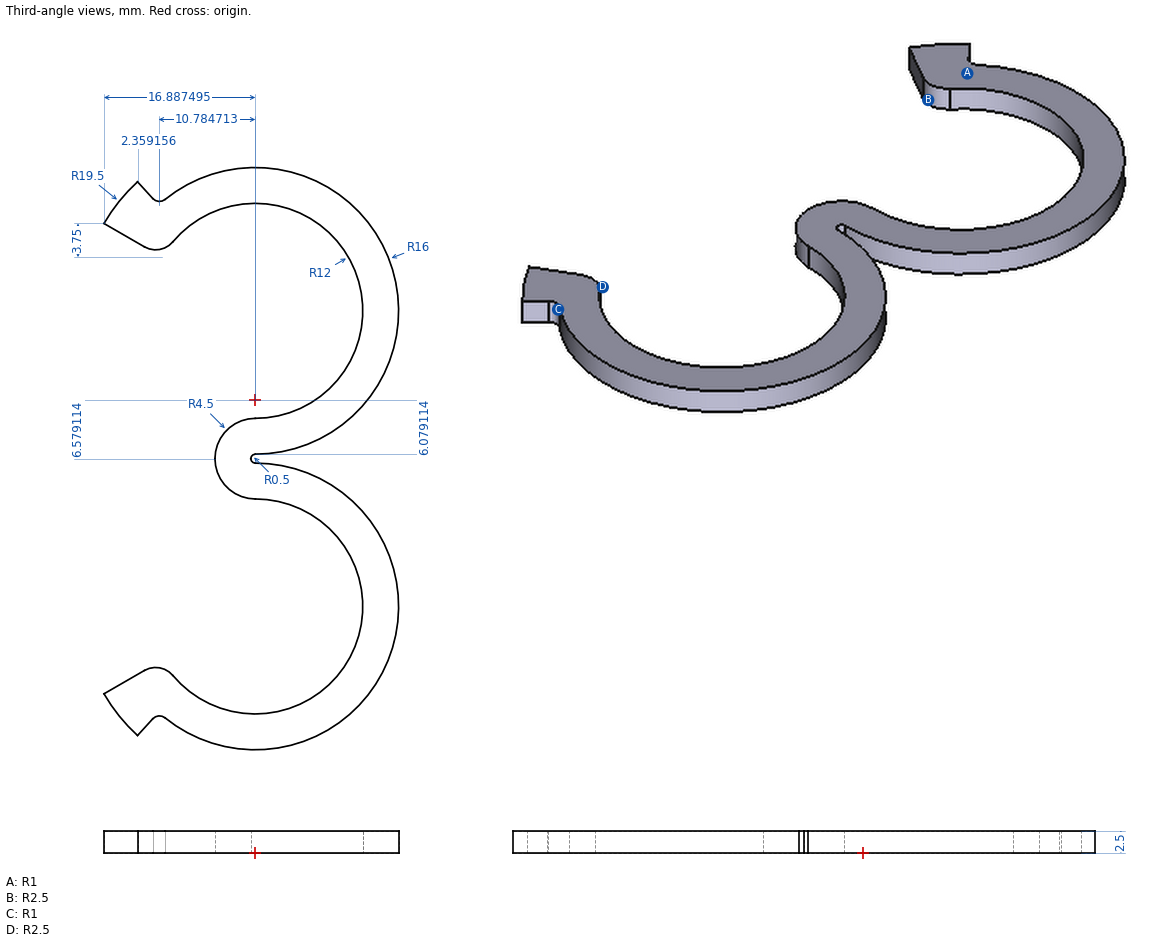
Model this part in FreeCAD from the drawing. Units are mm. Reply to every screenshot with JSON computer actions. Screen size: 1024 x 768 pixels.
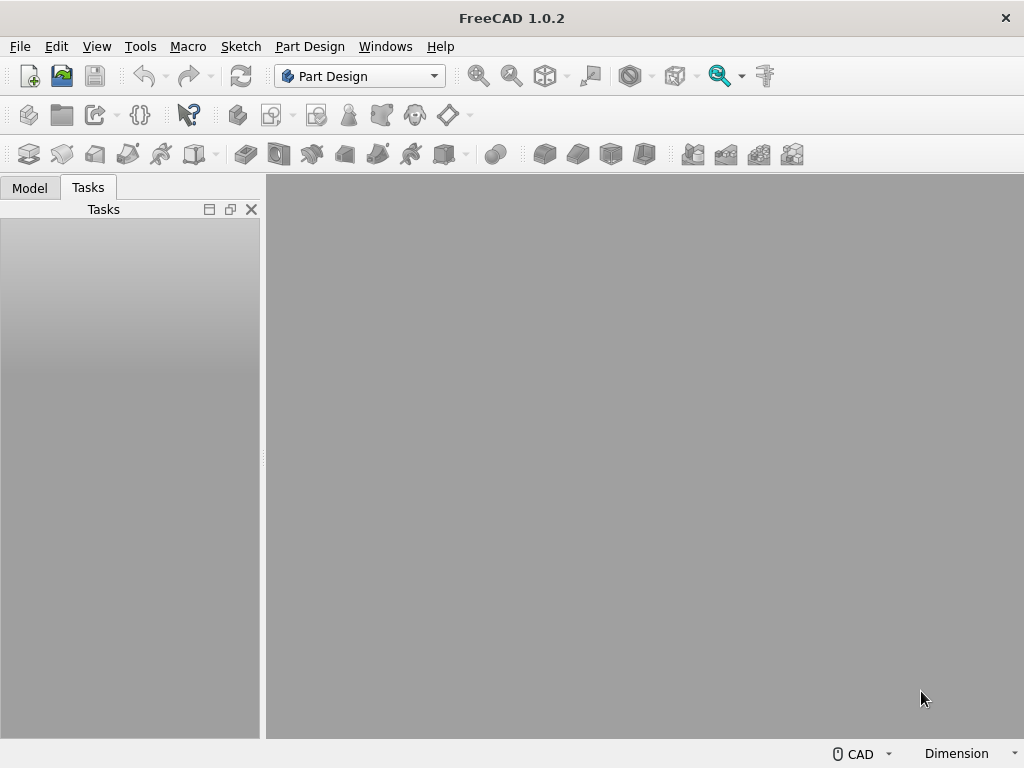
{"action": "left_click", "coordinate": [29, 76]}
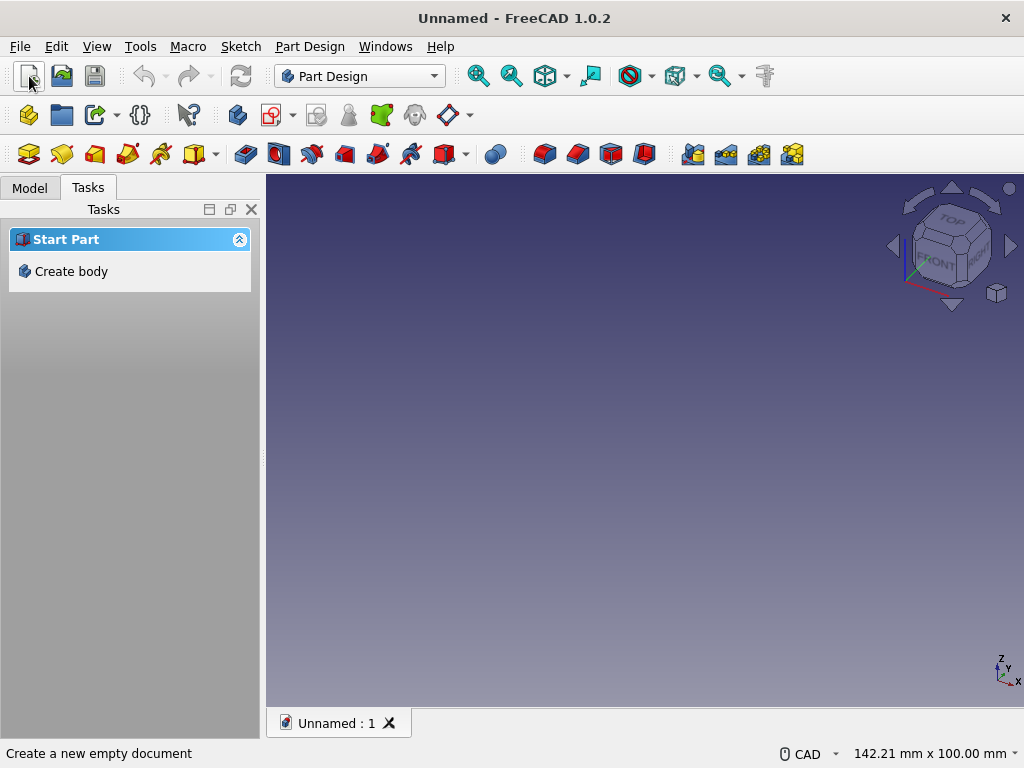
{"action": "left_click", "coordinate": [270, 116]}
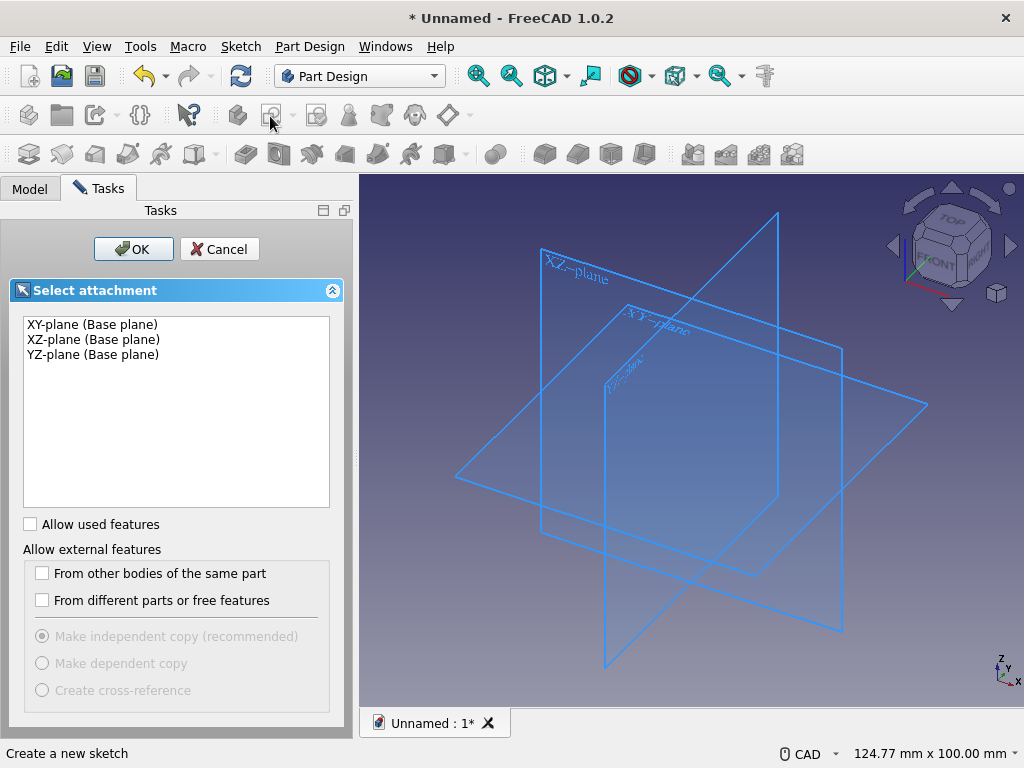
{"action": "left_click", "coordinate": [84, 324]}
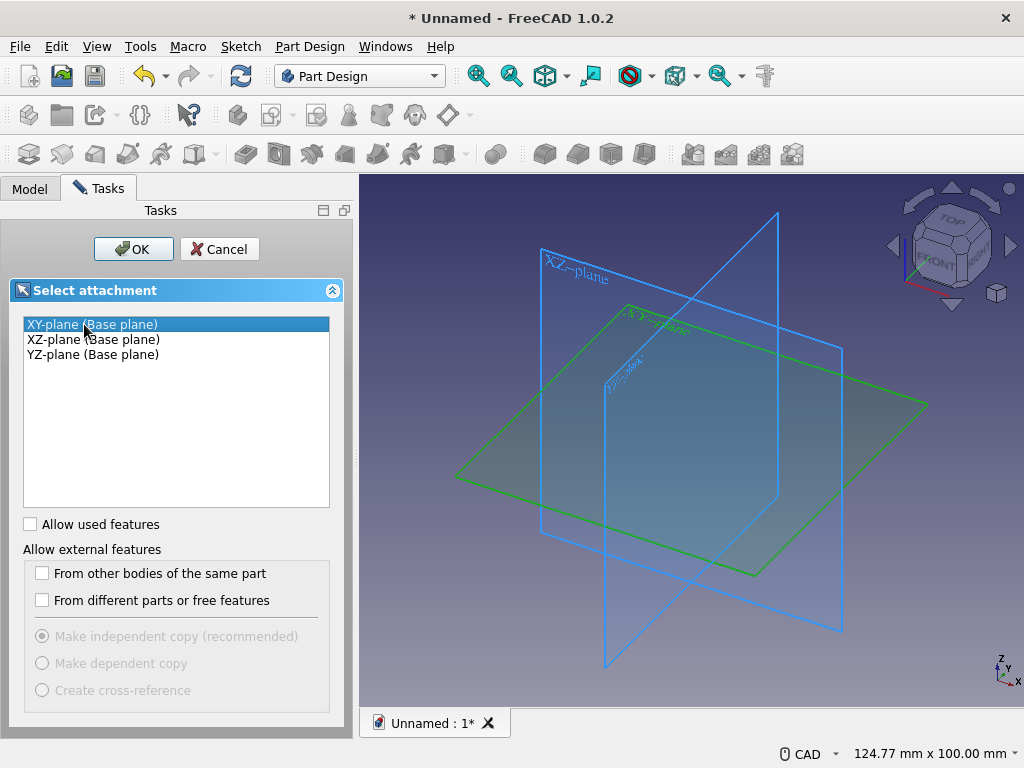
{"action": "left_click", "coordinate": [134, 249]}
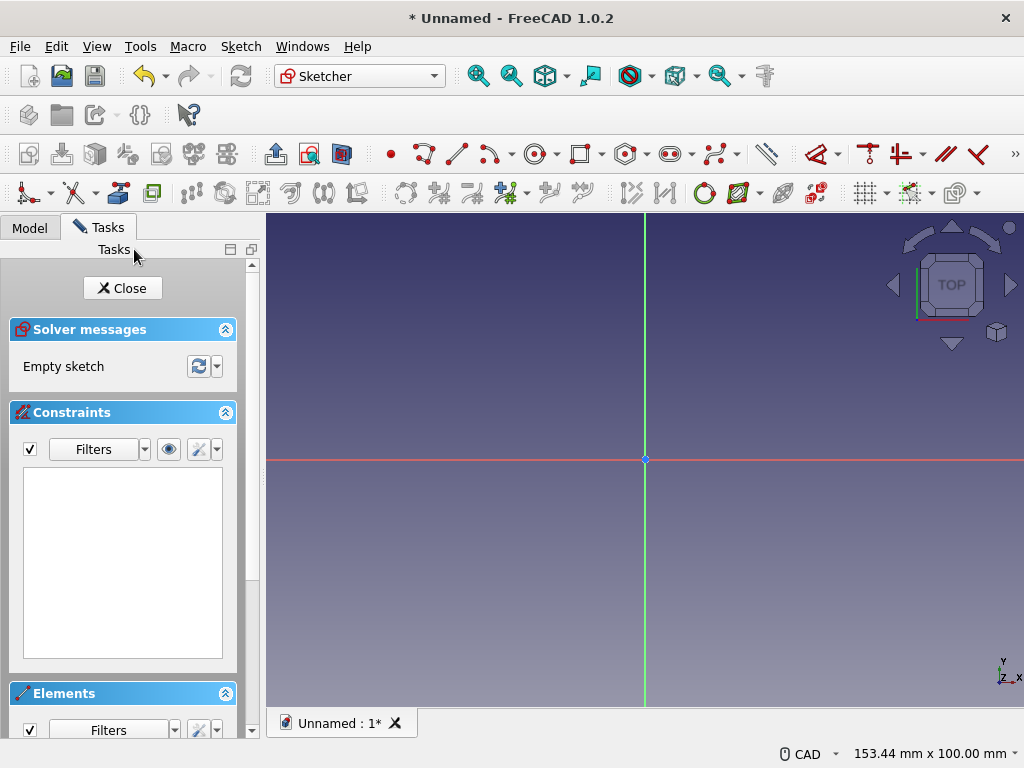
{"action": "scroll", "coordinate": [692, 380], "scroll_direction": "up", "scroll_amount": 4}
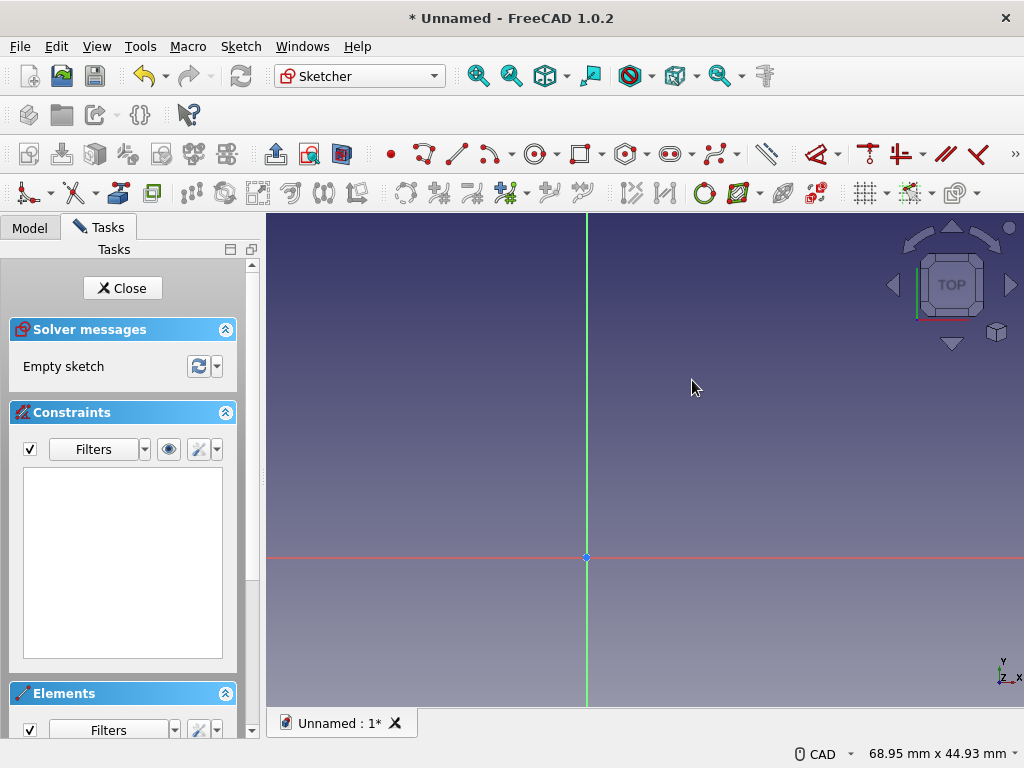
{"action": "left_click", "coordinate": [457, 154]}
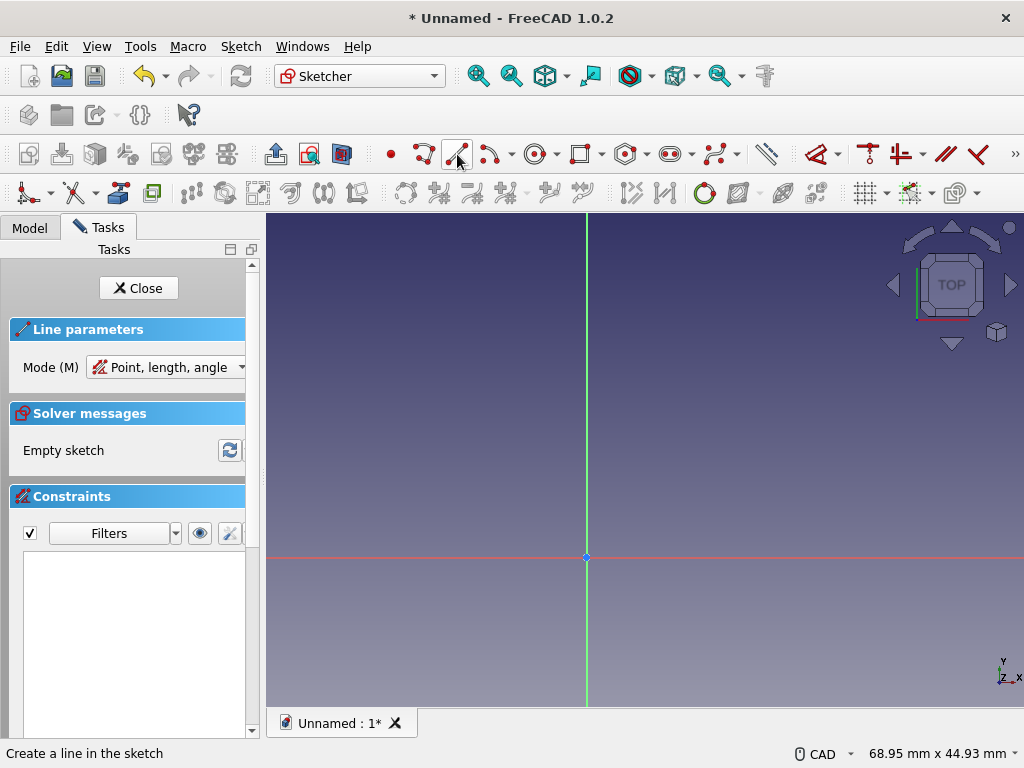
{"action": "left_click", "coordinate": [537, 630]}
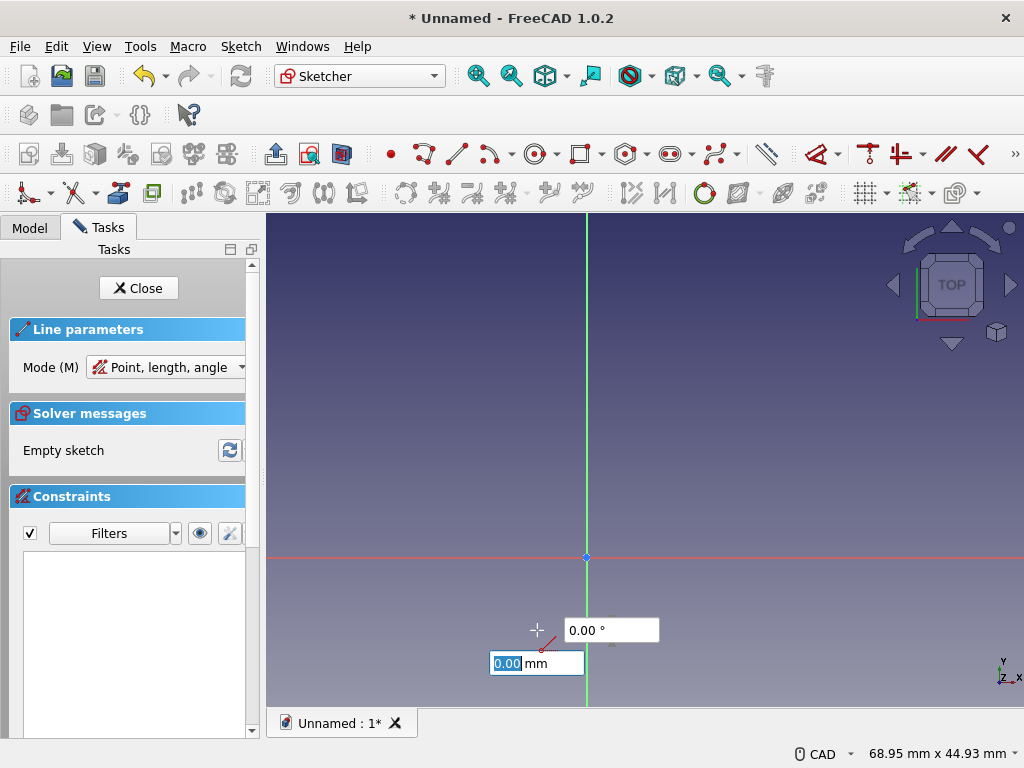
{"action": "scroll", "coordinate": [581, 630], "scroll_direction": "up", "scroll_amount": 6}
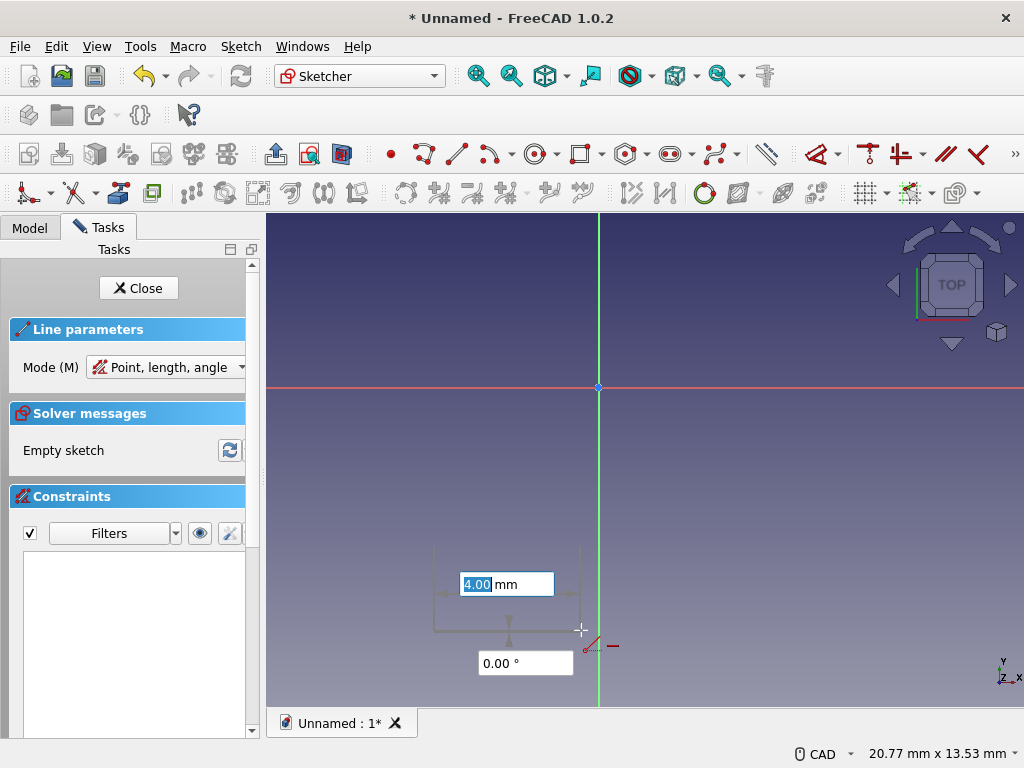
{"action": "left_click", "coordinate": [581, 628]}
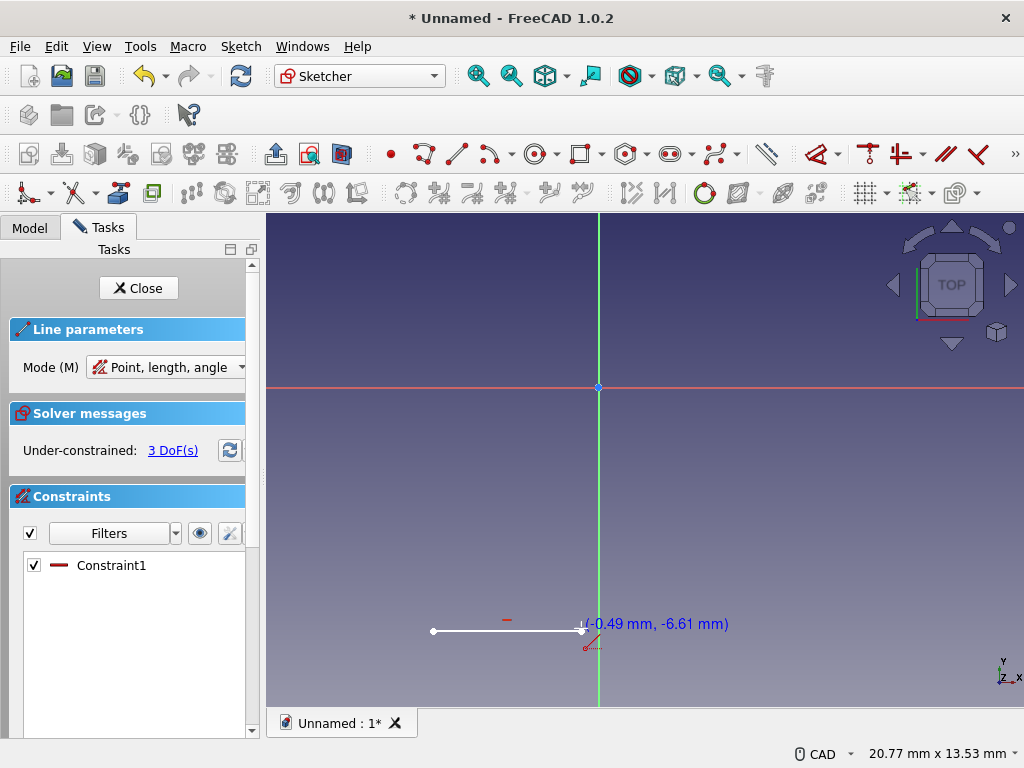
{"action": "scroll", "coordinate": [582, 631], "scroll_direction": "down", "scroll_amount": 6}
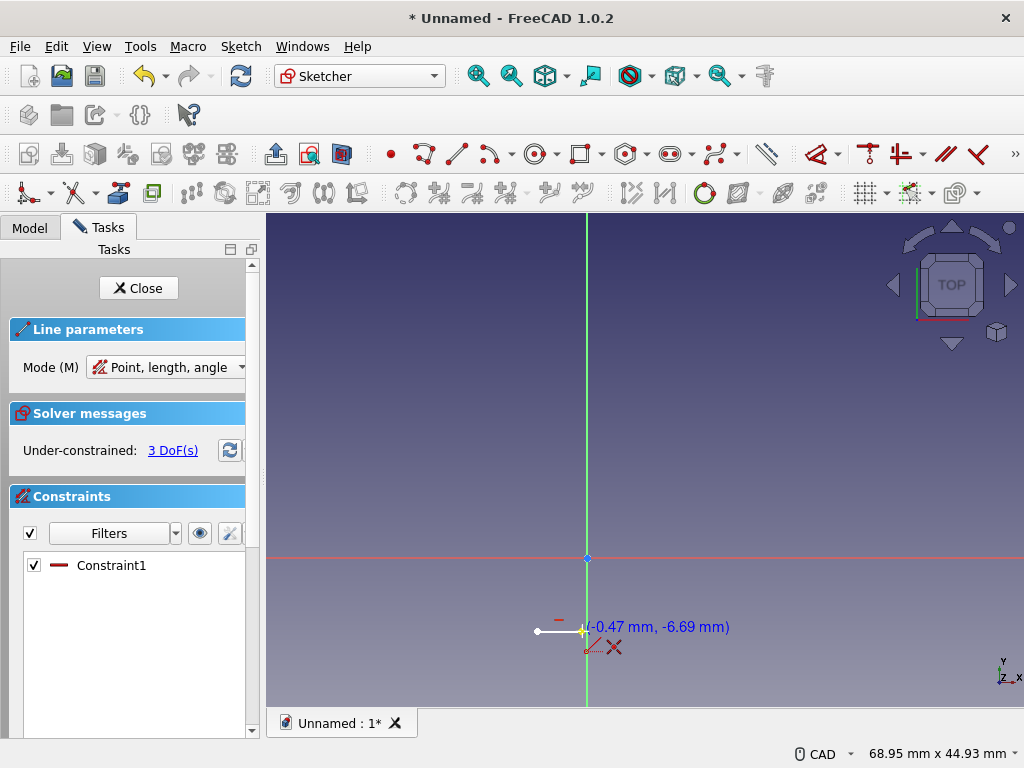
{"action": "left_click", "coordinate": [469, 319]}
{"action": "left_click", "coordinate": [443, 291]}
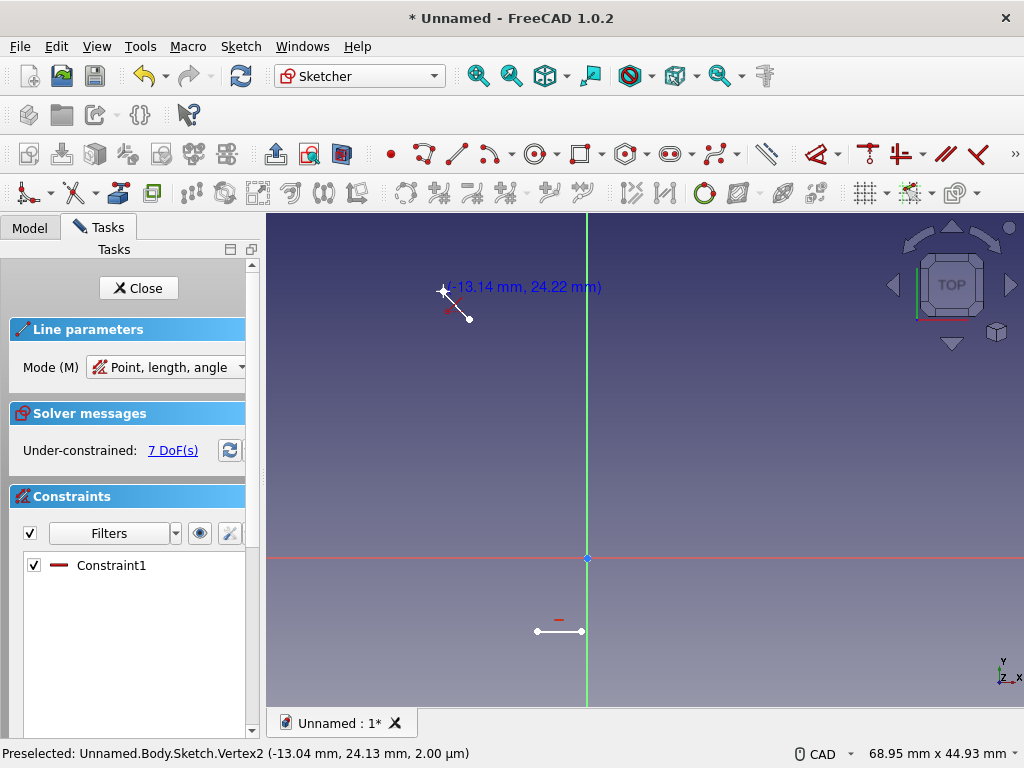
{"action": "left_click", "coordinate": [402, 342]}
{"action": "left_click", "coordinate": [473, 383]}